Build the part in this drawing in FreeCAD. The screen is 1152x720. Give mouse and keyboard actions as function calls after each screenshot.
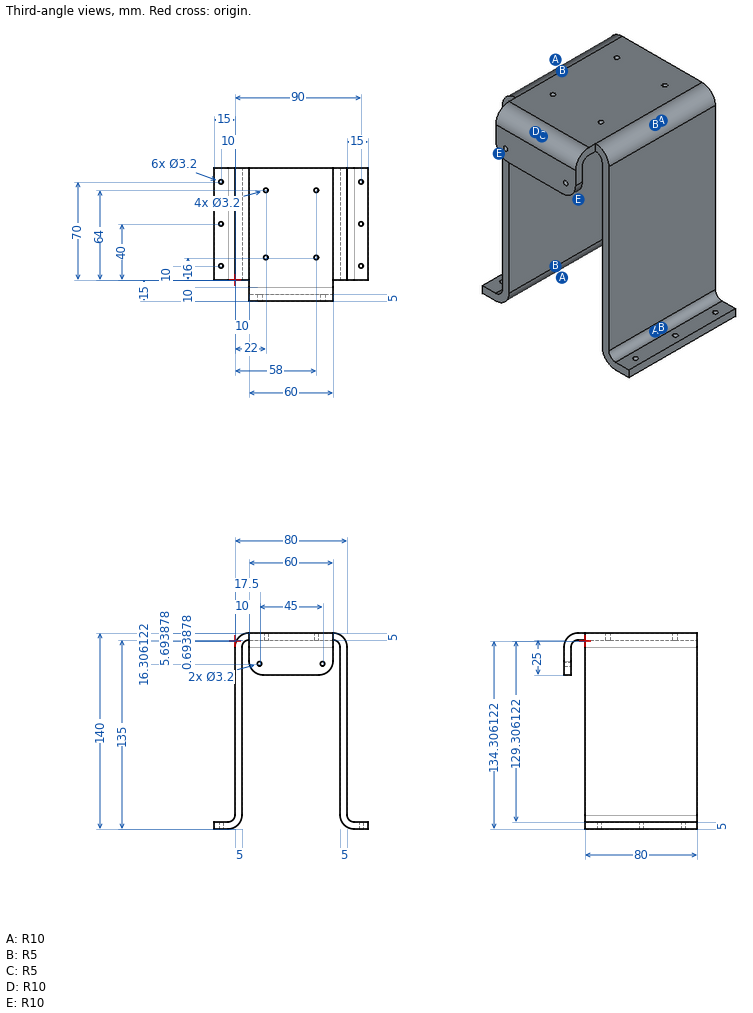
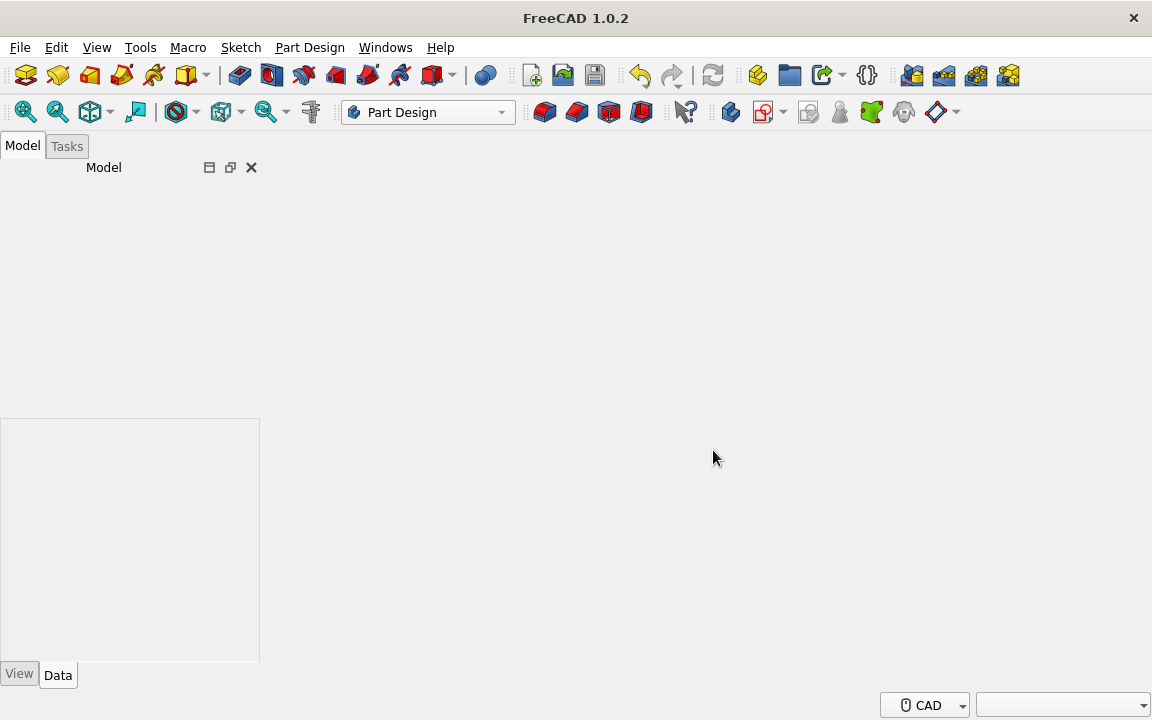
click(532, 76)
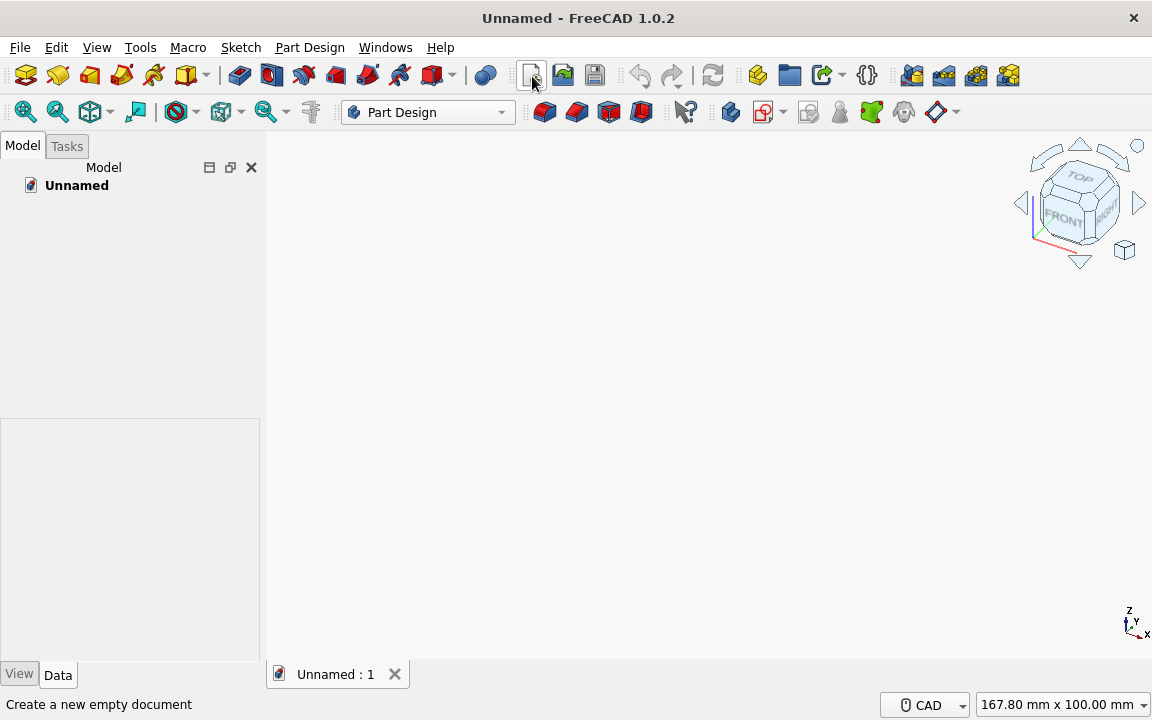
click(764, 112)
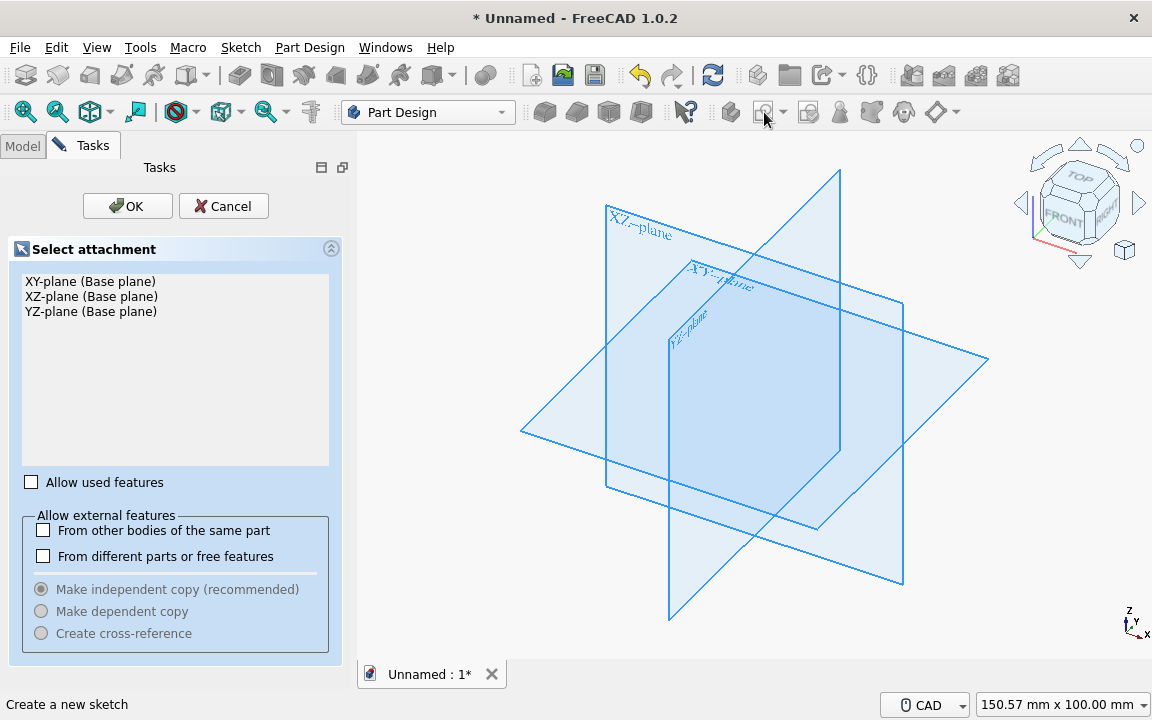
click(82, 296)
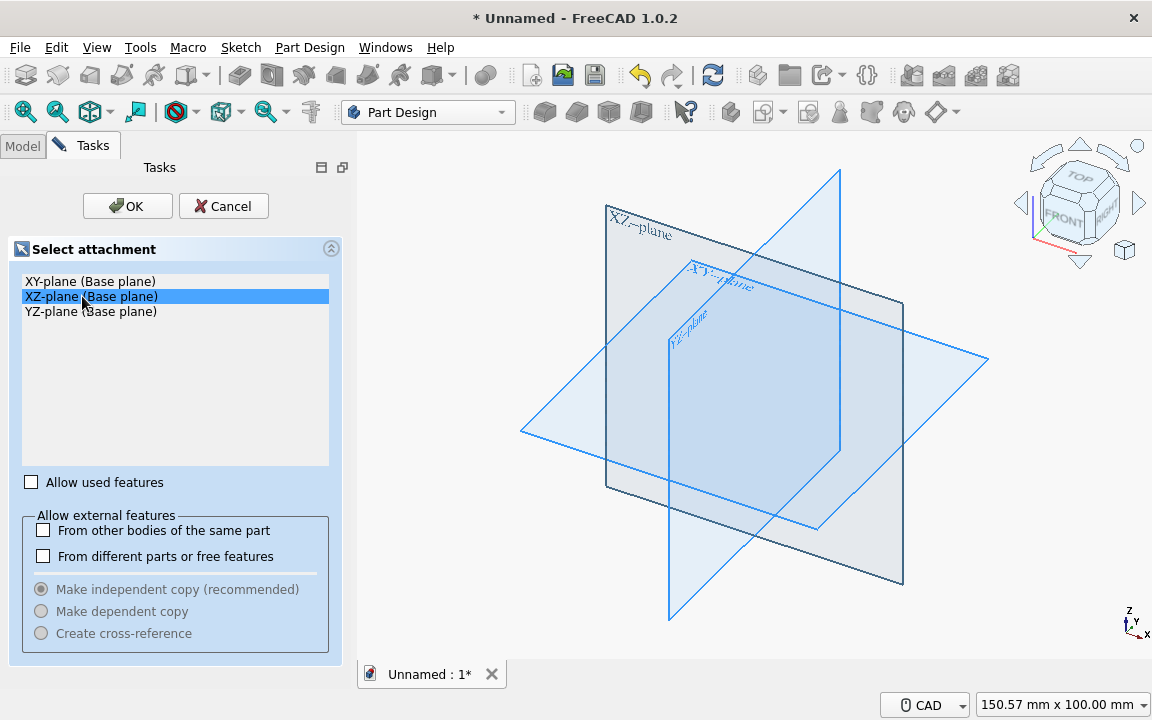
click(128, 206)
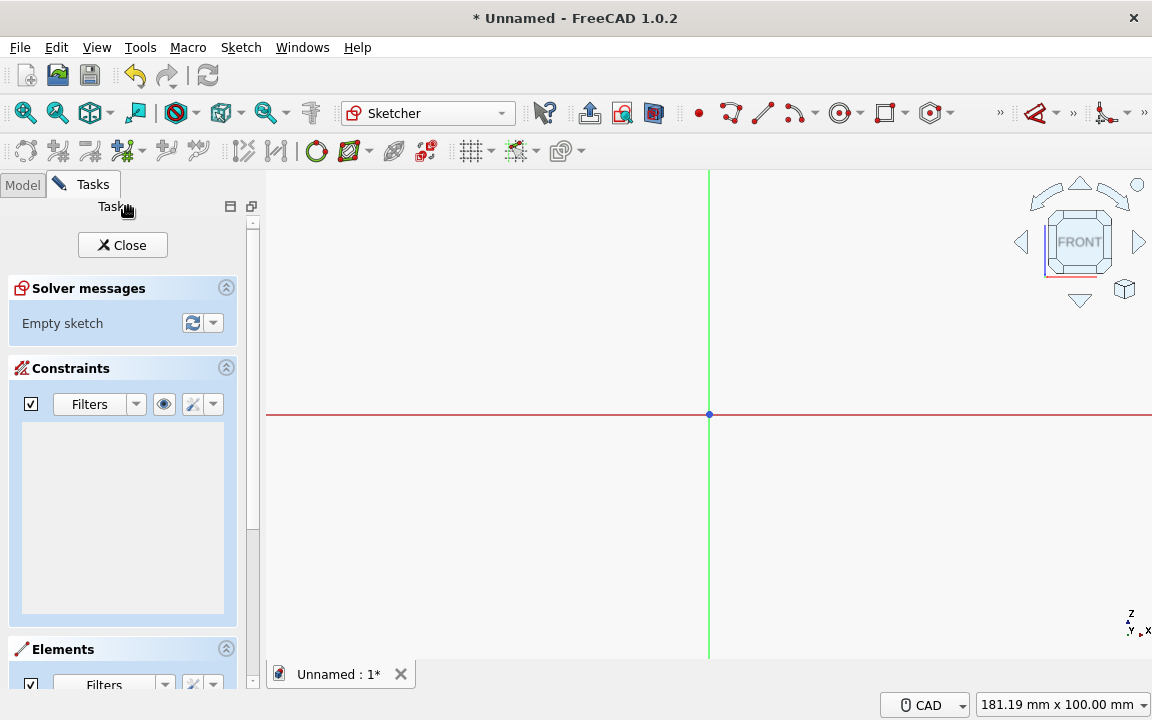
scroll(425, 198, down, 4)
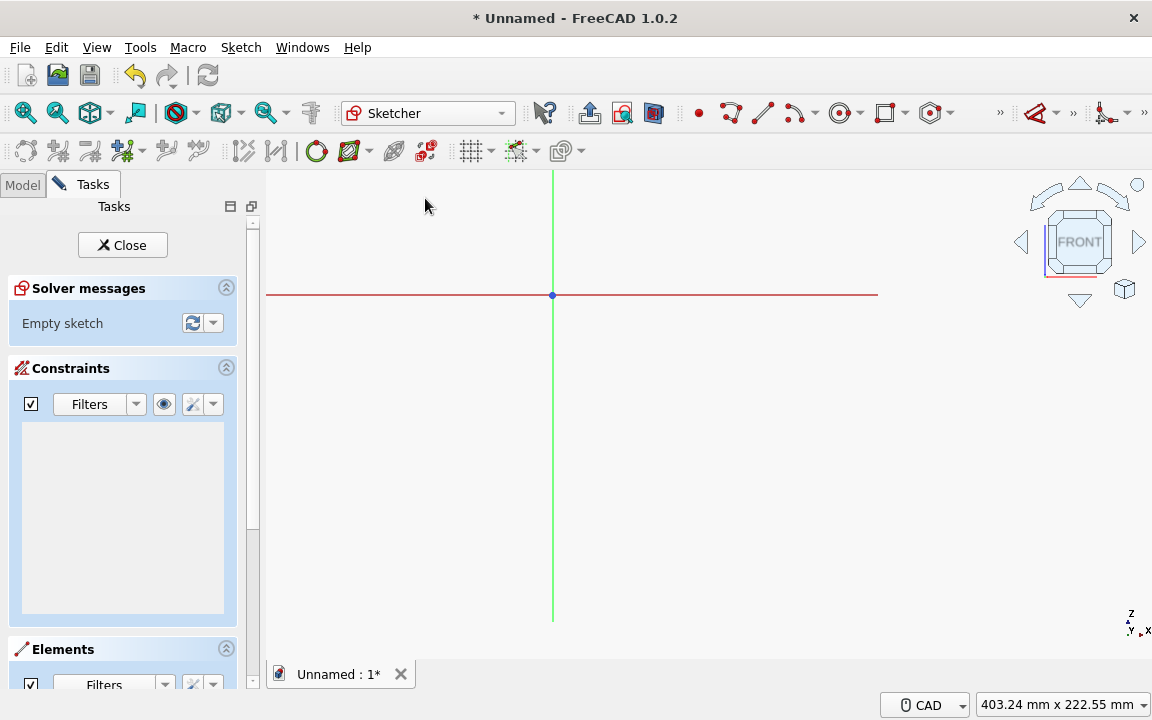
click(732, 114)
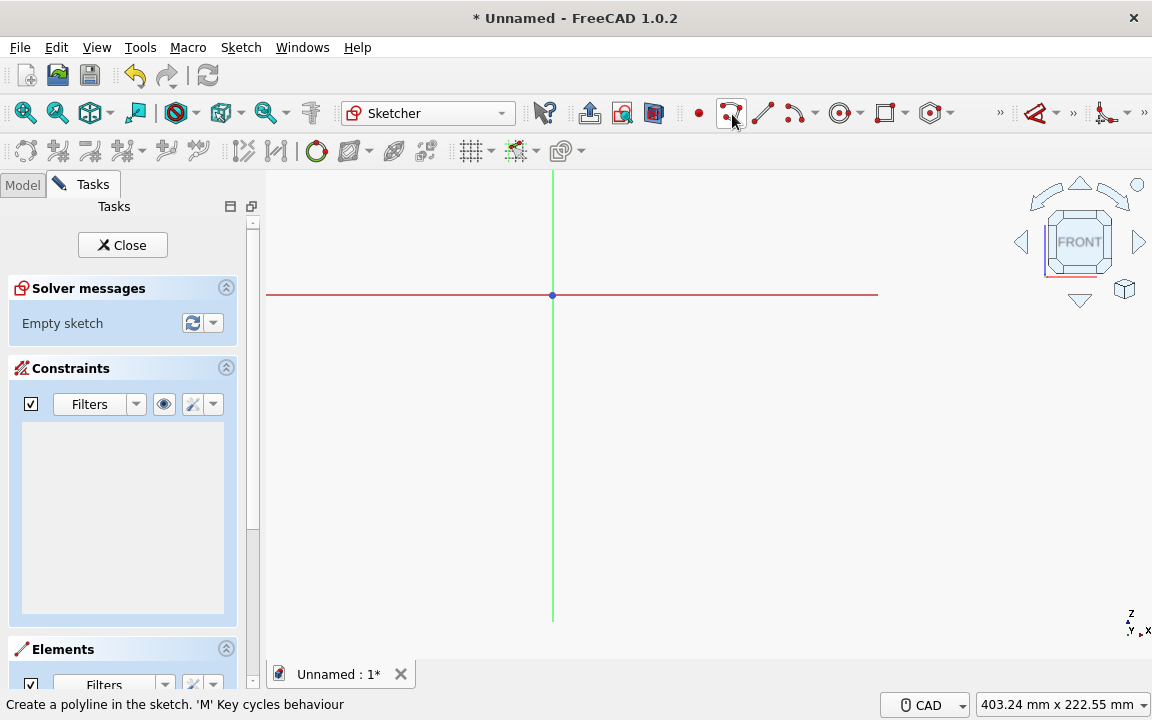
scroll(564, 294, up, 12)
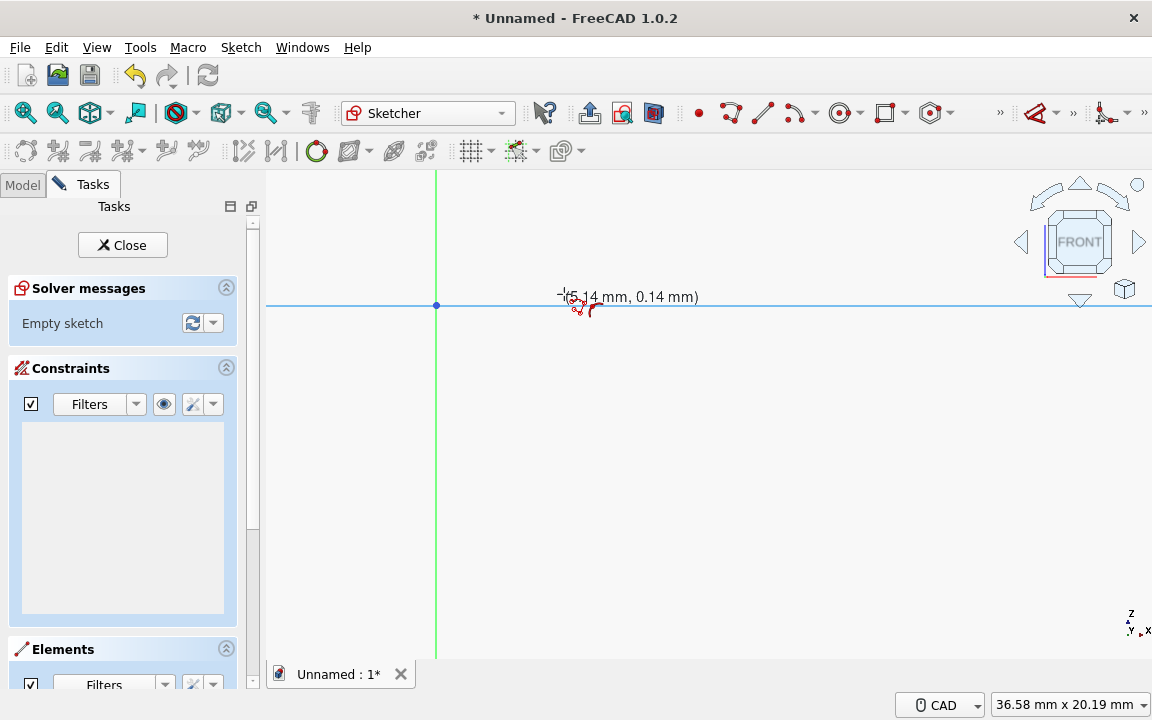
click(557, 289)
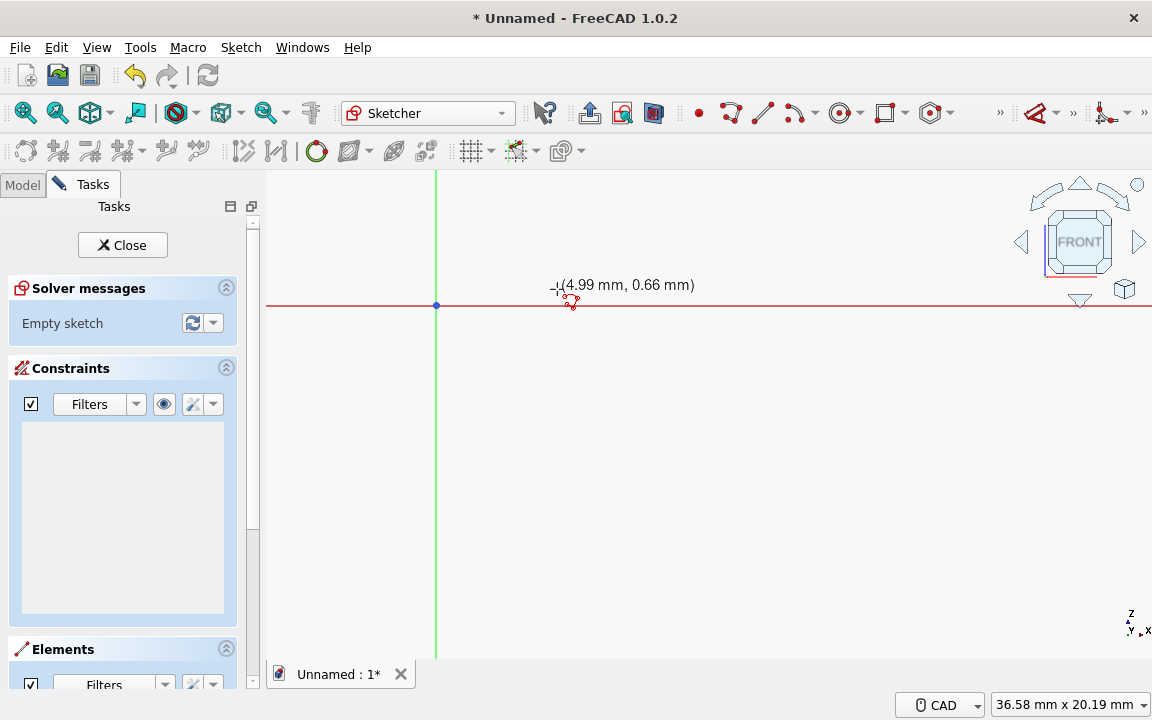
scroll(564, 270, down, 12)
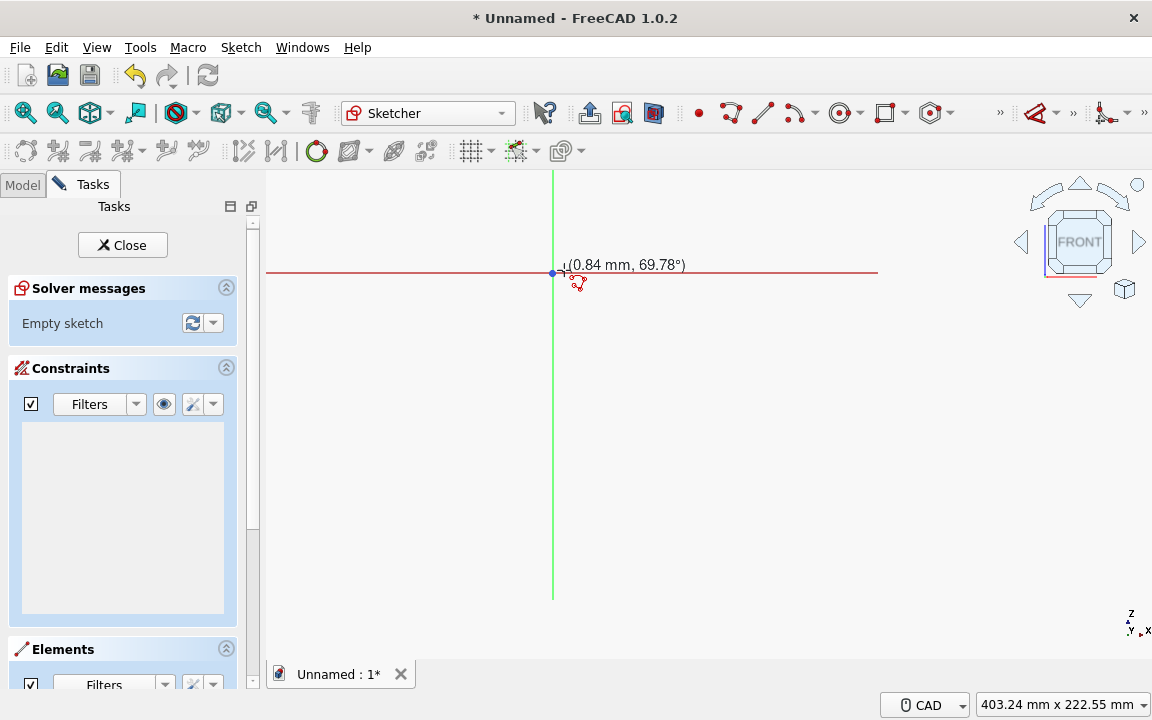
scroll(564, 569, up, 2)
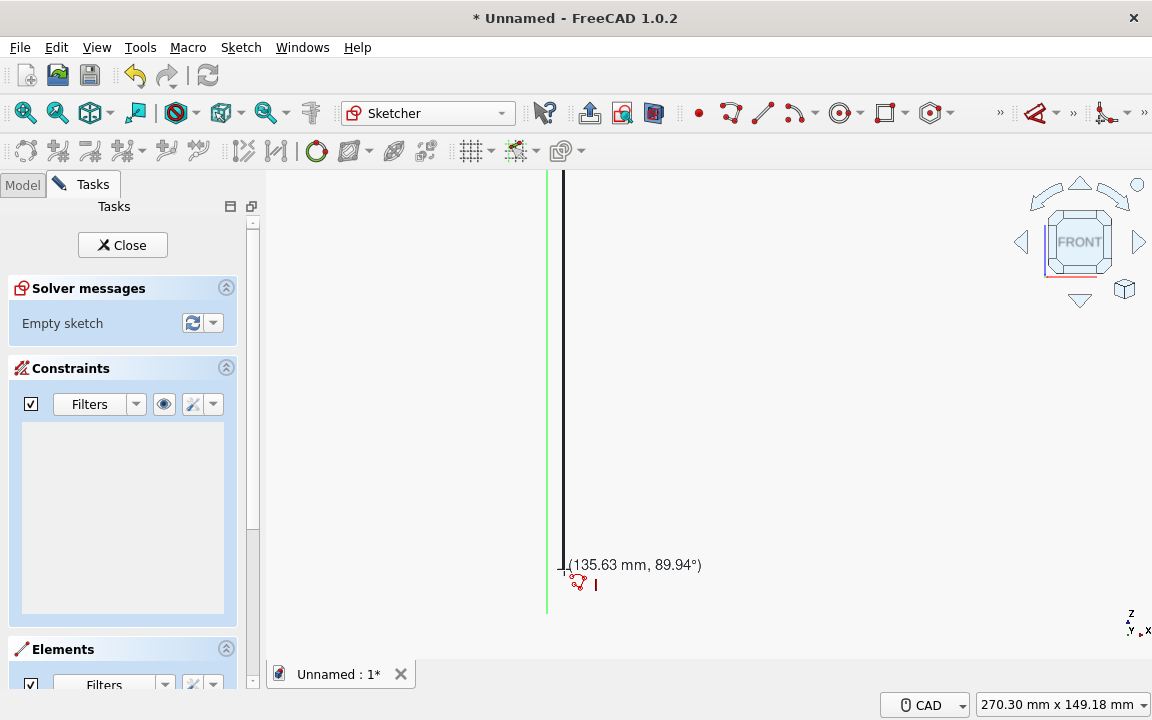
click(563, 568)
click(547, 568)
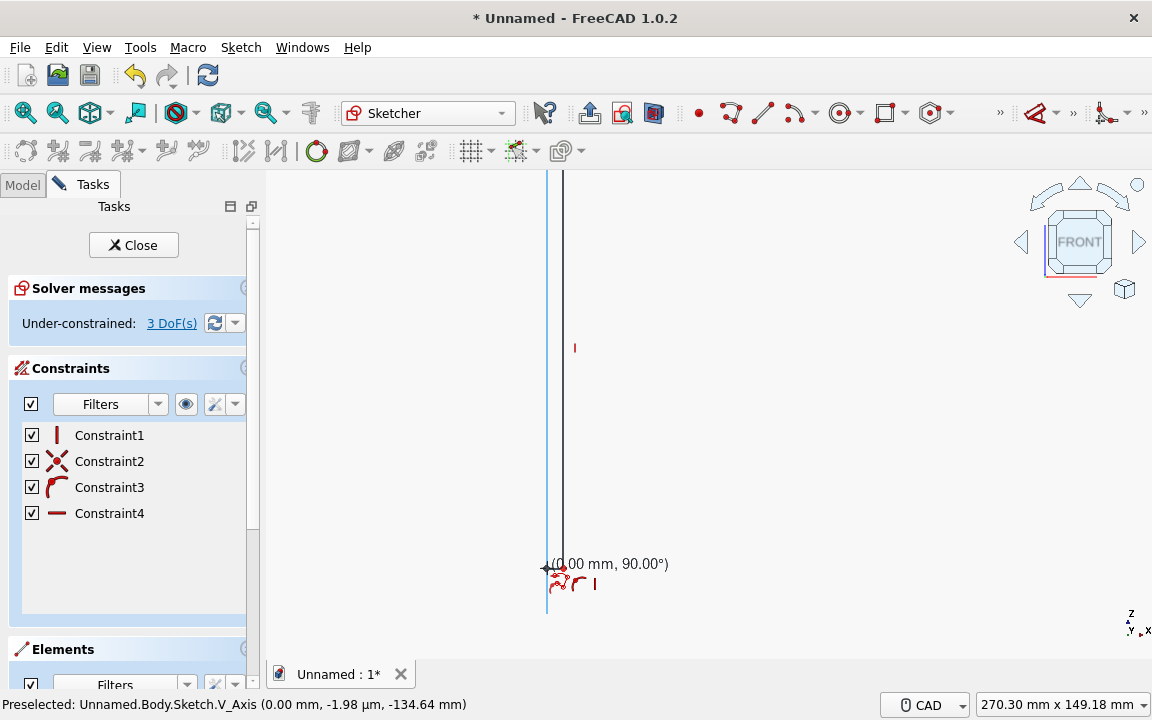
scroll(564, 569, down, 2)